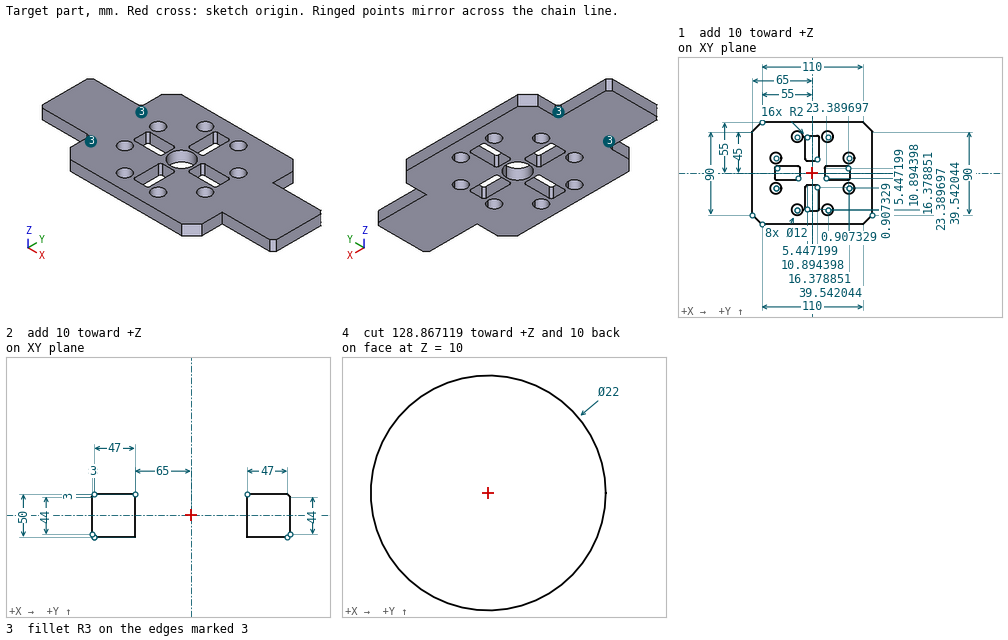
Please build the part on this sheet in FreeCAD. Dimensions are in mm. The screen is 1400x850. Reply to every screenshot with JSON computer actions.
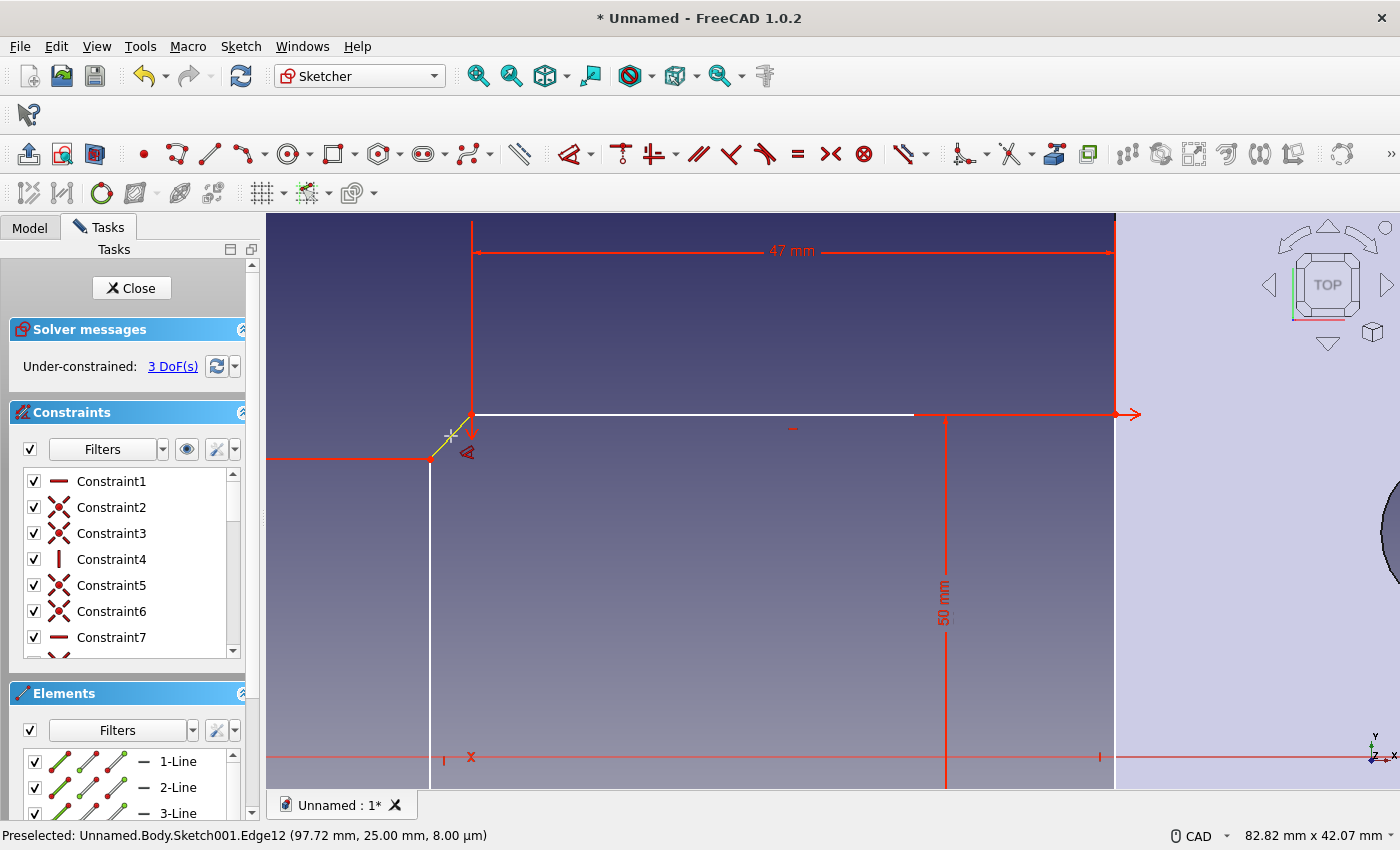
{"action": "left_click", "coordinate": [451, 437]}
{"action": "left_click", "coordinate": [451, 381]}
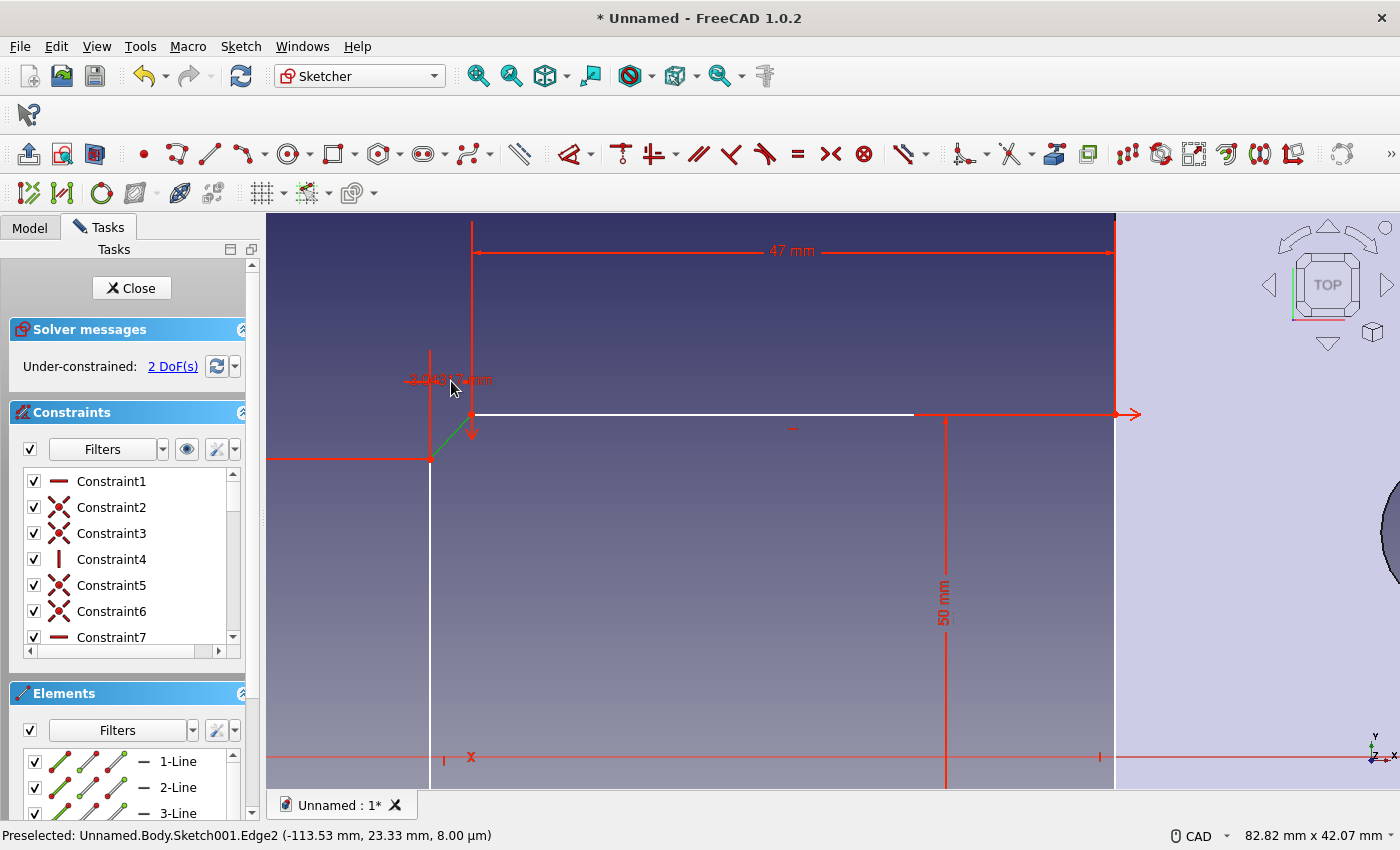
{"action": "type", "text": "3"}
{"action": "key", "text": "Return"}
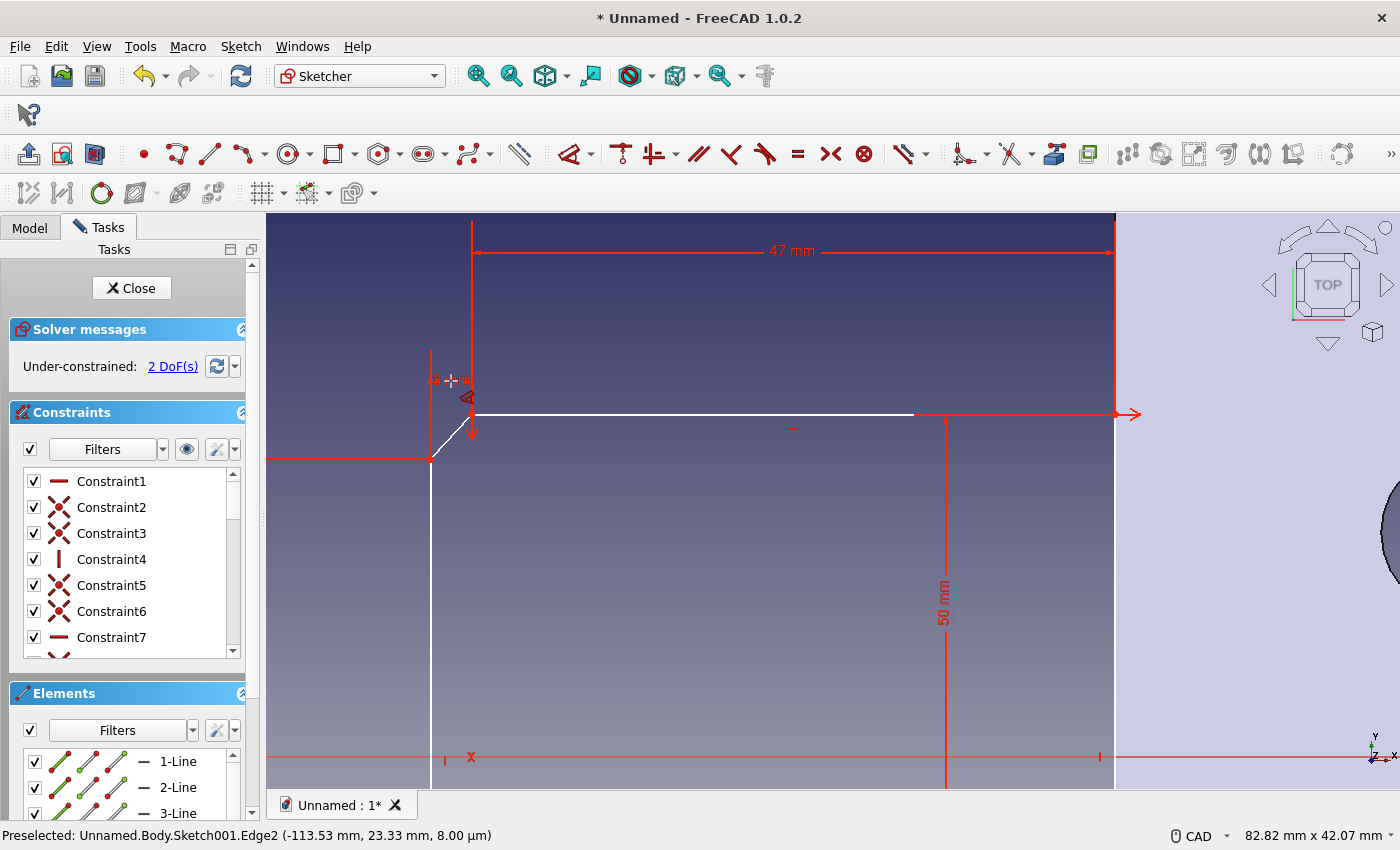
{"action": "left_click", "coordinate": [459, 428]}
{"action": "left_click", "coordinate": [397, 437]}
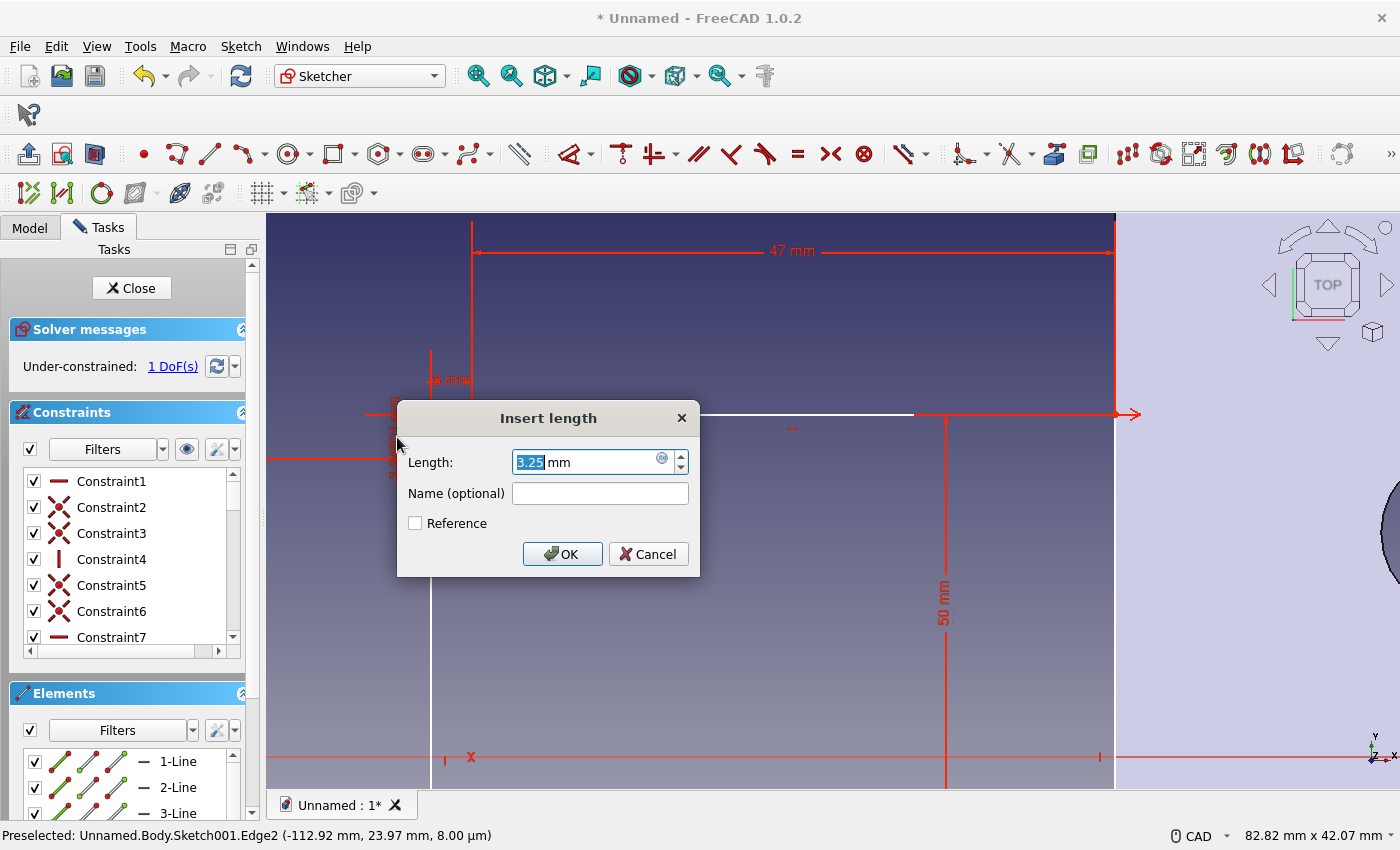
{"action": "type", "text": "3"}
{"action": "key", "text": "Return"}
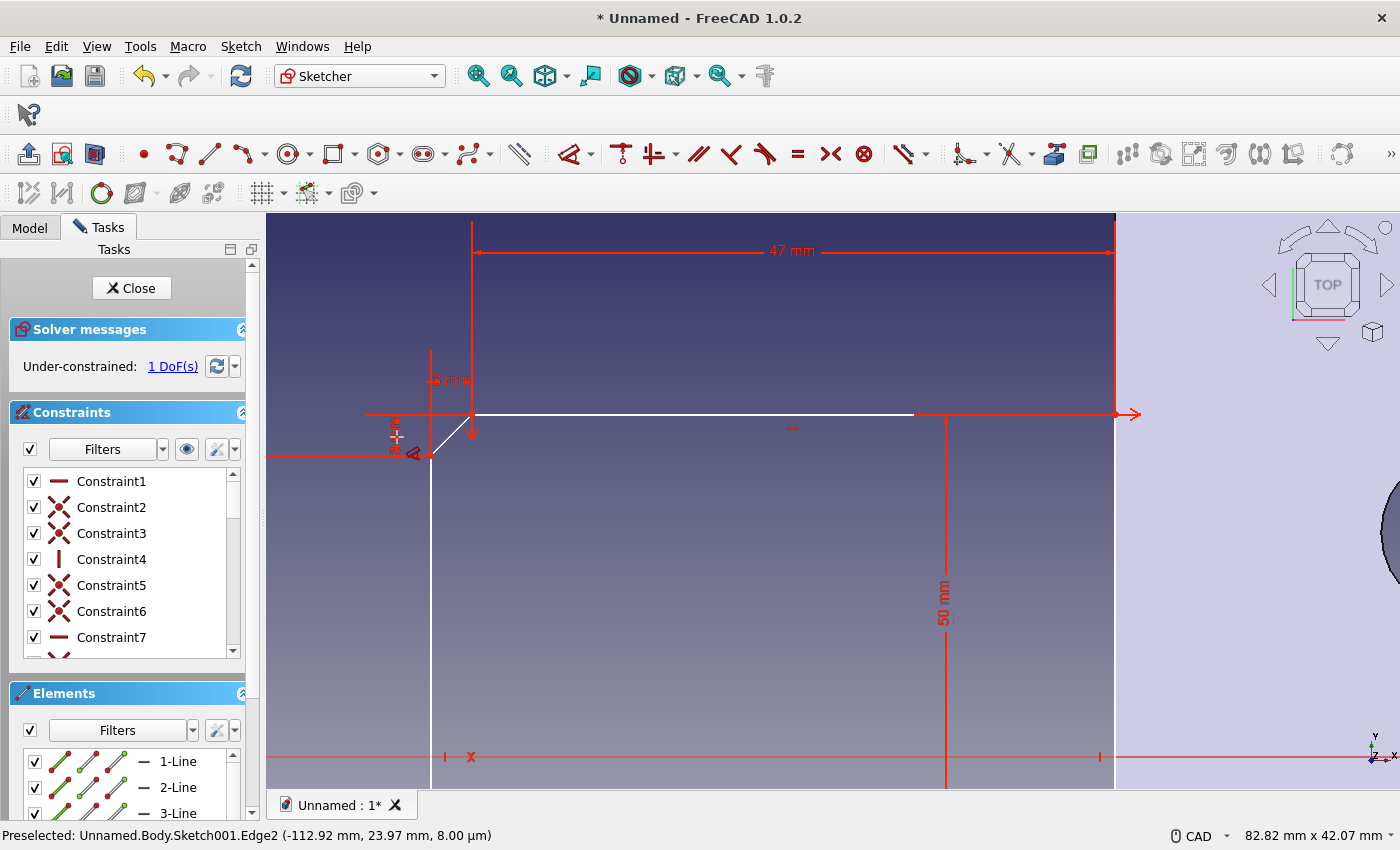
{"action": "scroll", "coordinate": [451, 436], "scroll_direction": "down", "scroll_amount": 8}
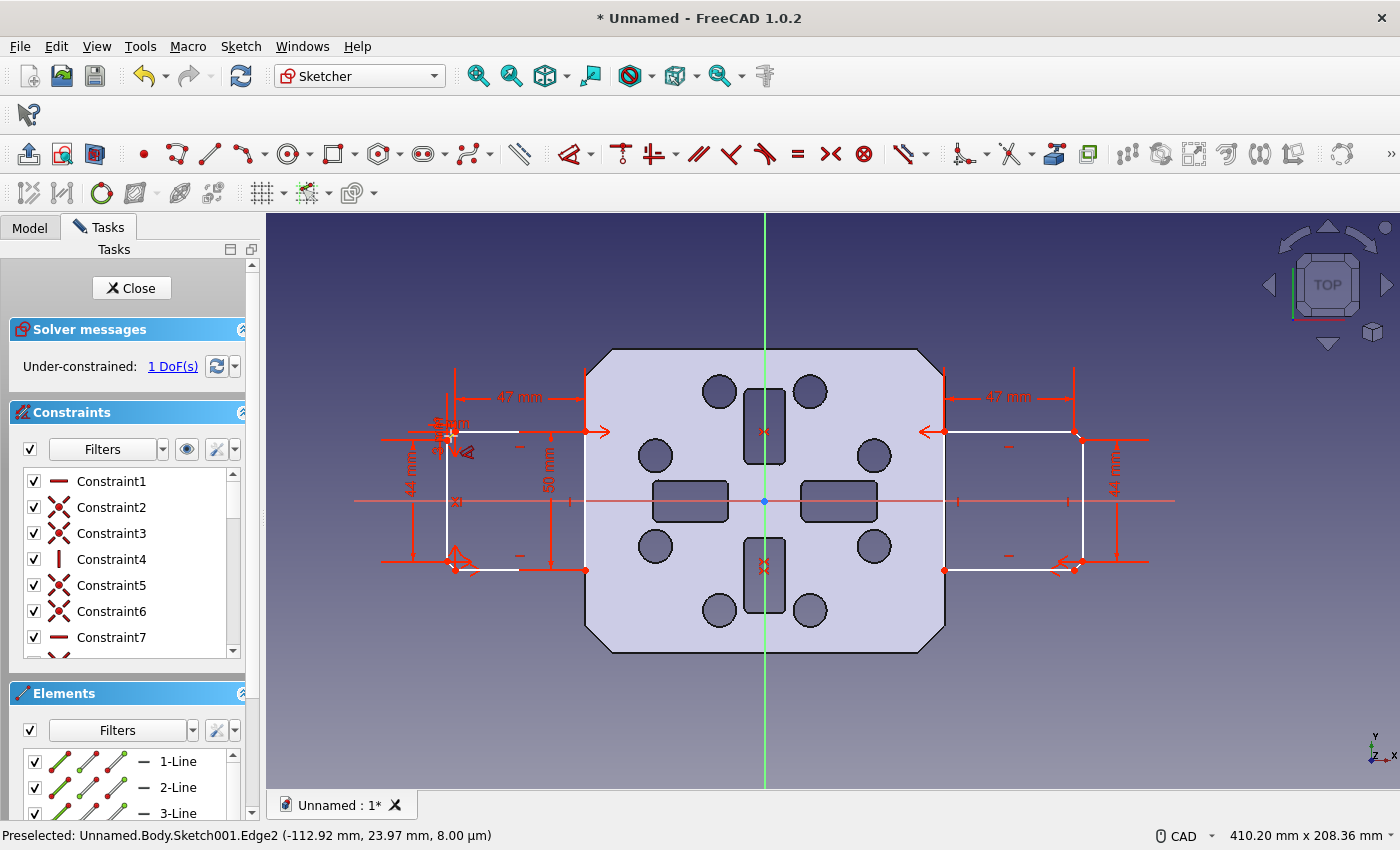
{"action": "left_click", "coordinate": [585, 432]}
{"action": "left_click", "coordinate": [675, 398]}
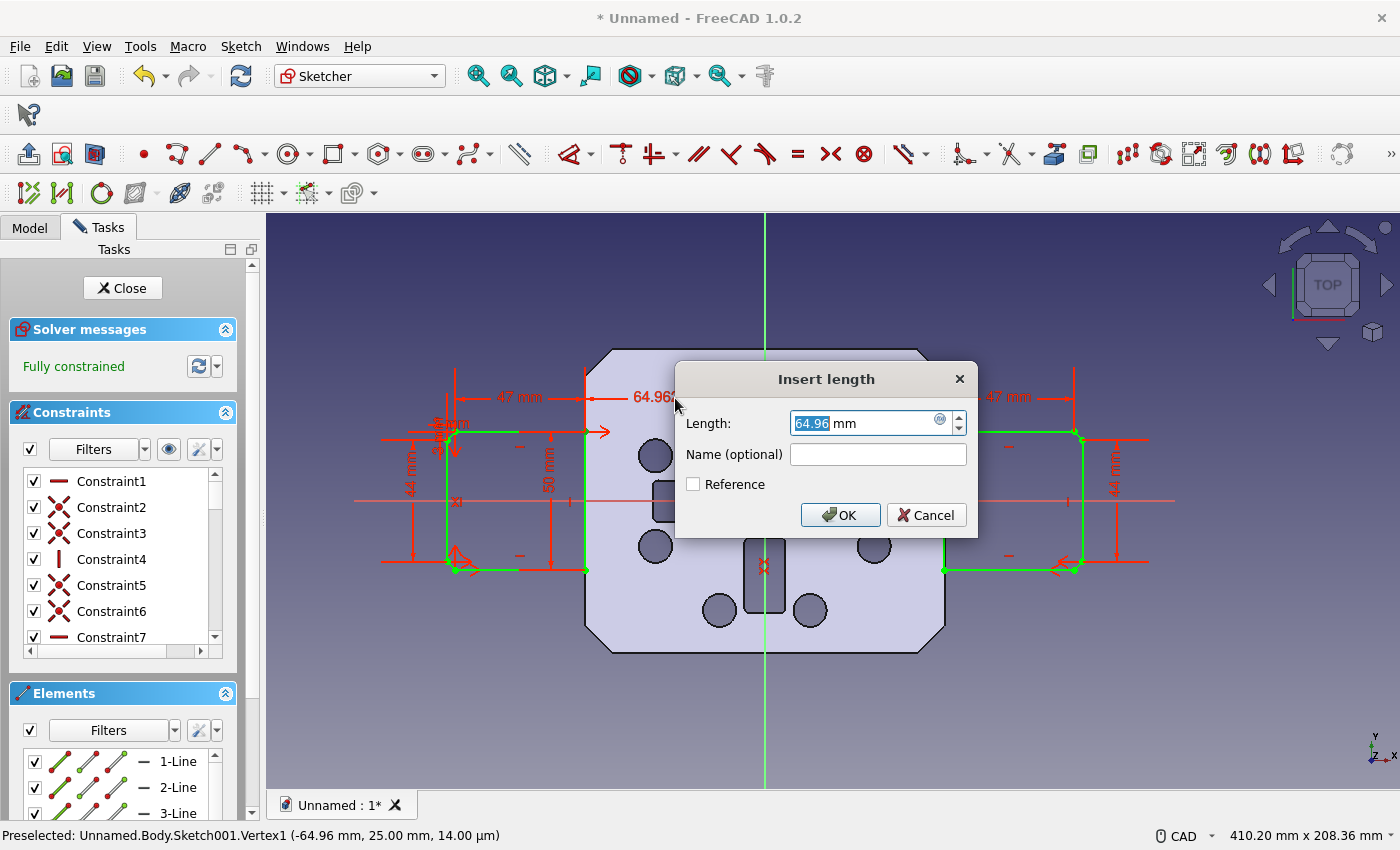
{"action": "type", "text": "65"}
{"action": "key", "text": "Return"}
{"action": "key", "text": "Escape"}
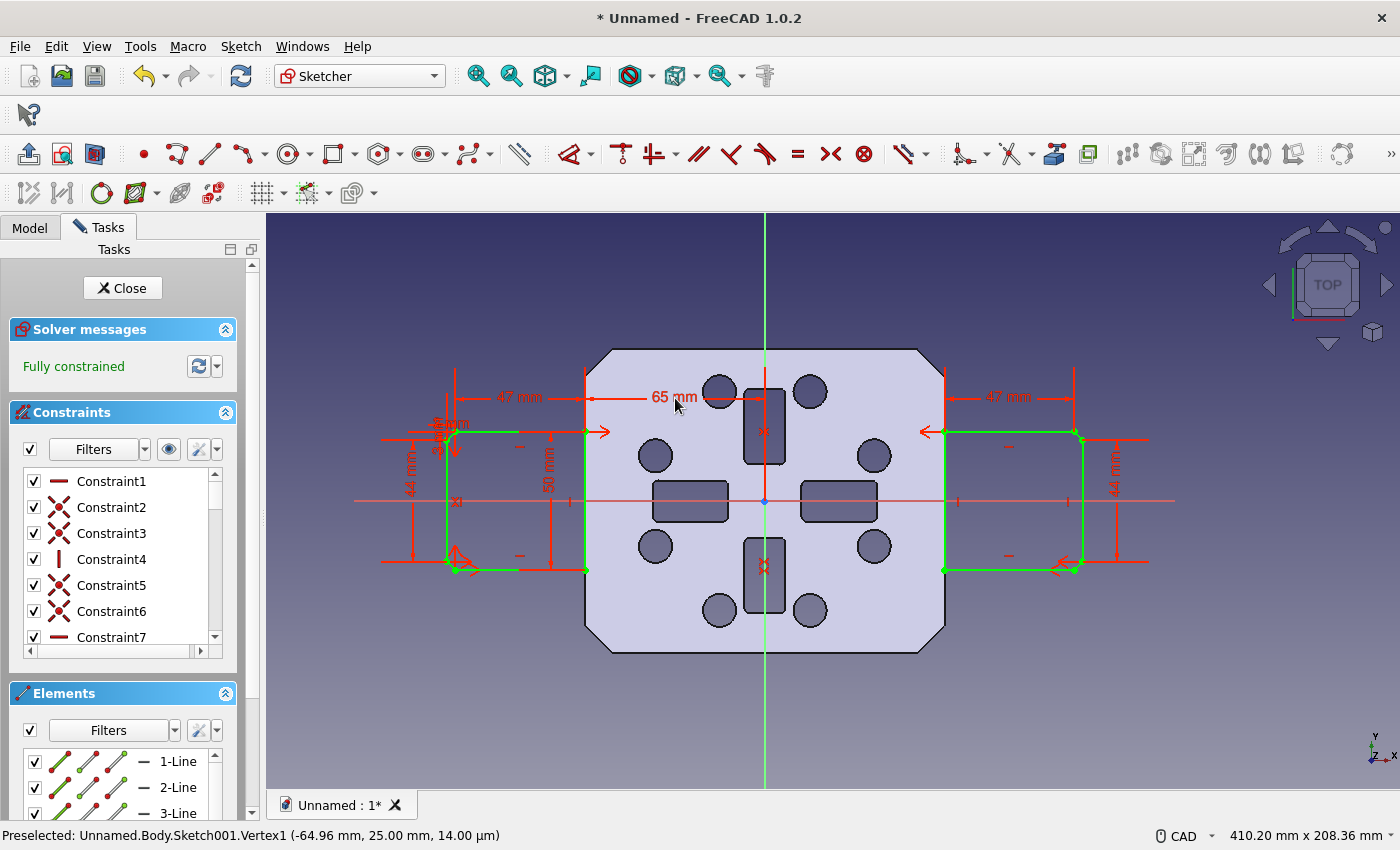
{"action": "left_click", "coordinate": [123, 288]}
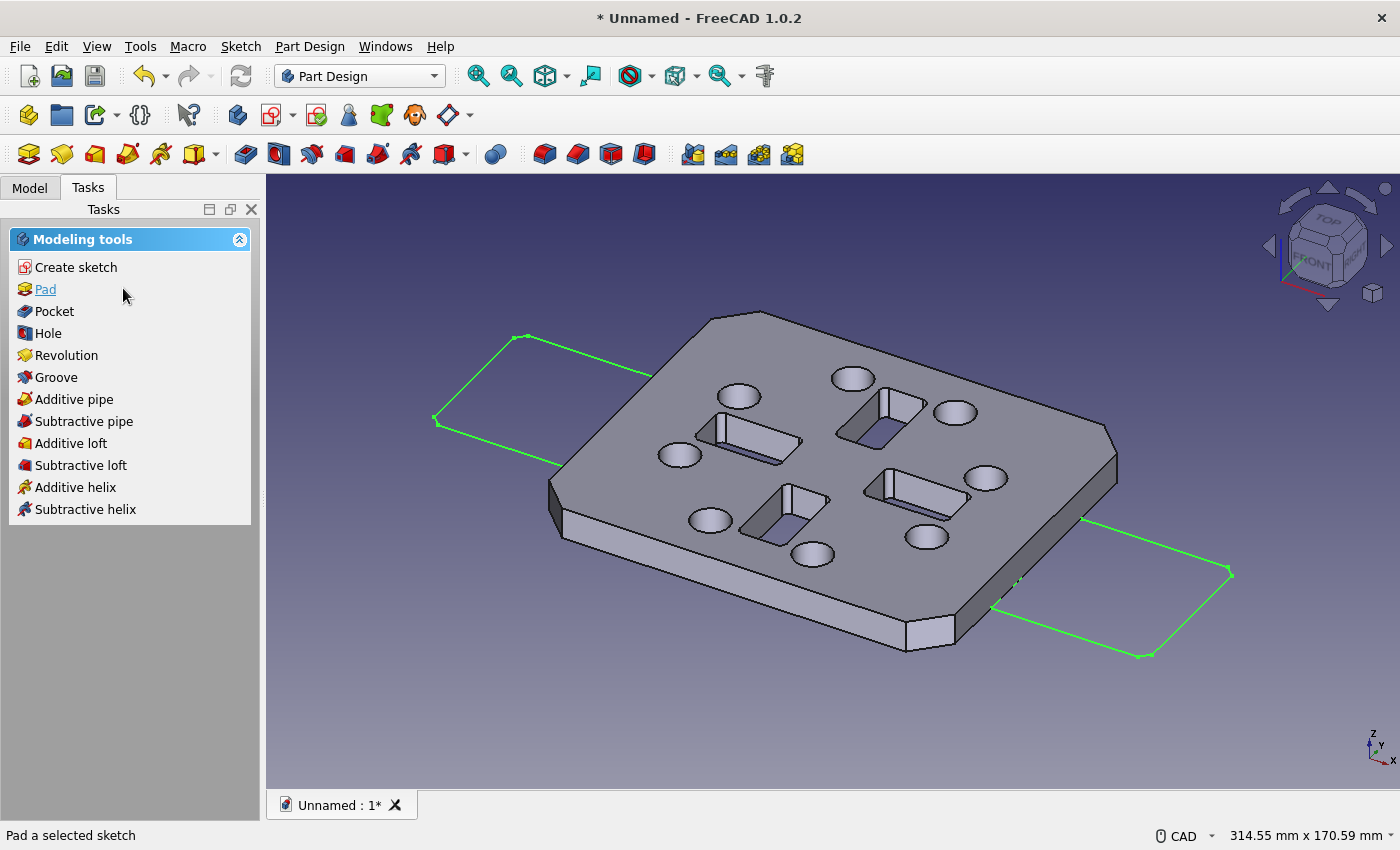
{"action": "left_click", "coordinate": [29, 154]}